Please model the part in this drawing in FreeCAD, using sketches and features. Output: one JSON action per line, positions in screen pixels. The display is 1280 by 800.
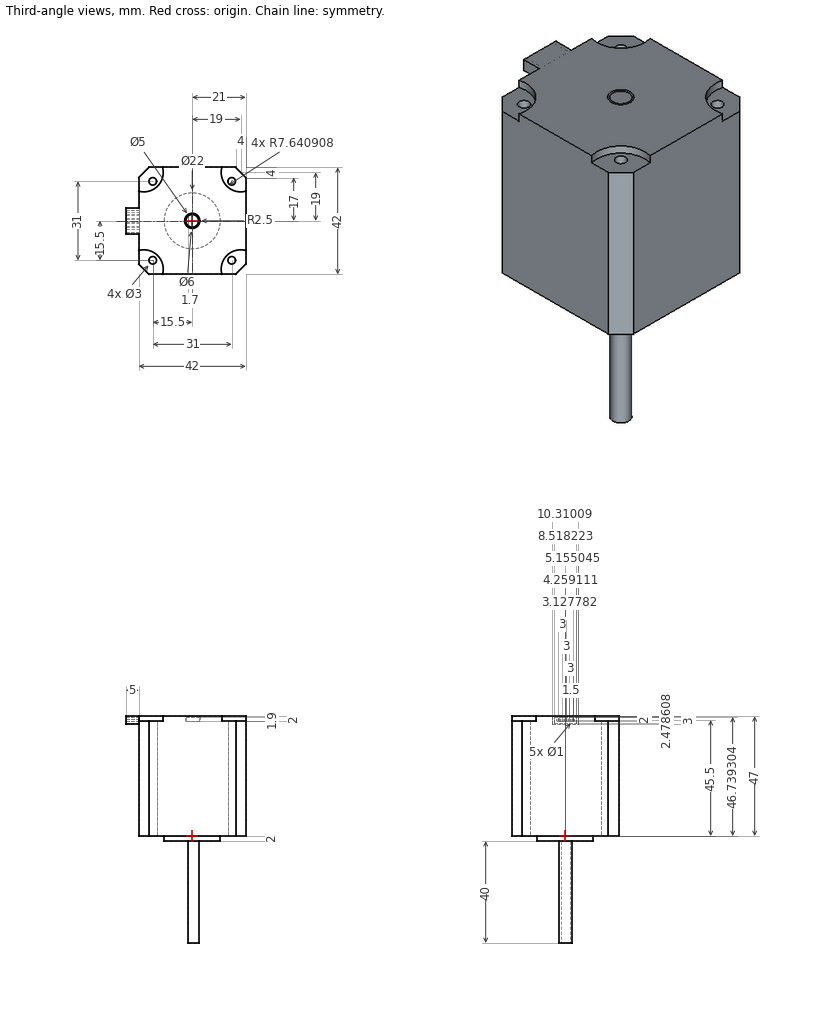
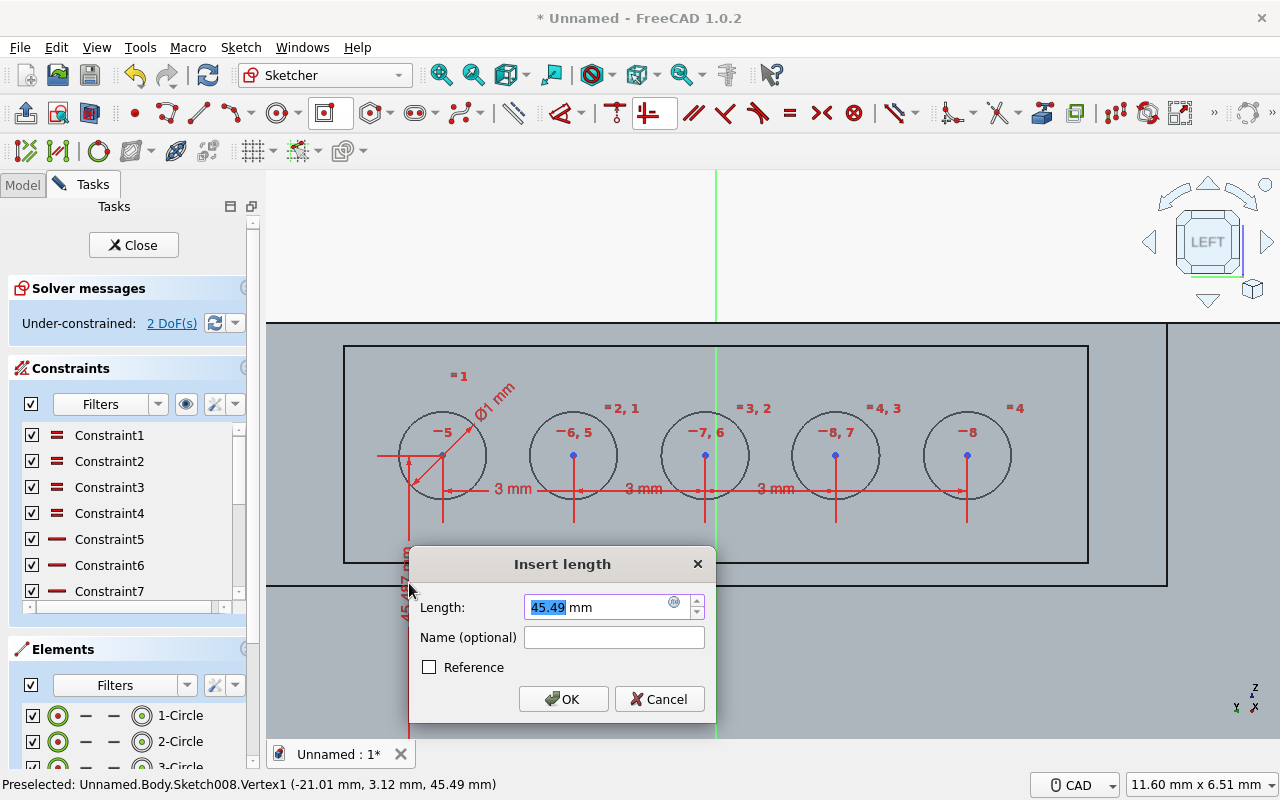
{"action": "type", "text": "45.5"}
{"action": "key", "text": "Return"}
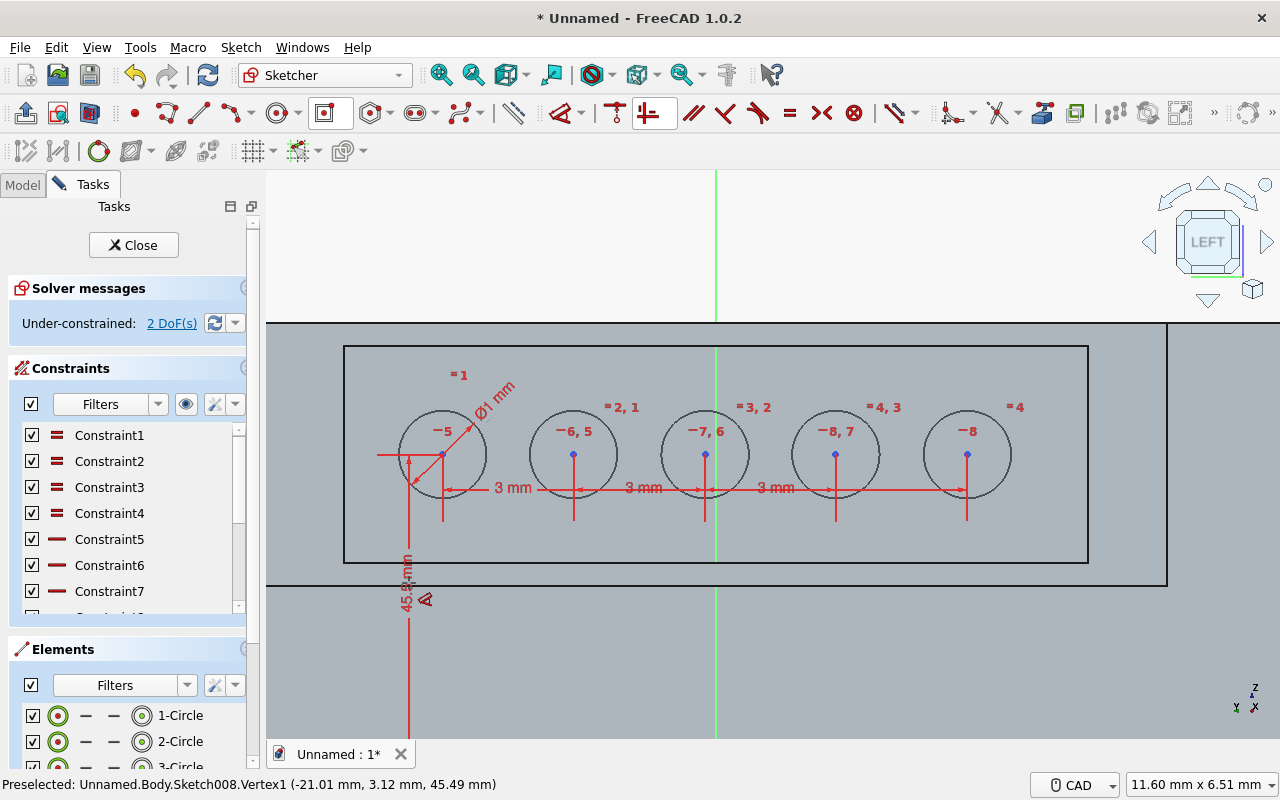
{"action": "left_click", "coordinate": [443, 455]}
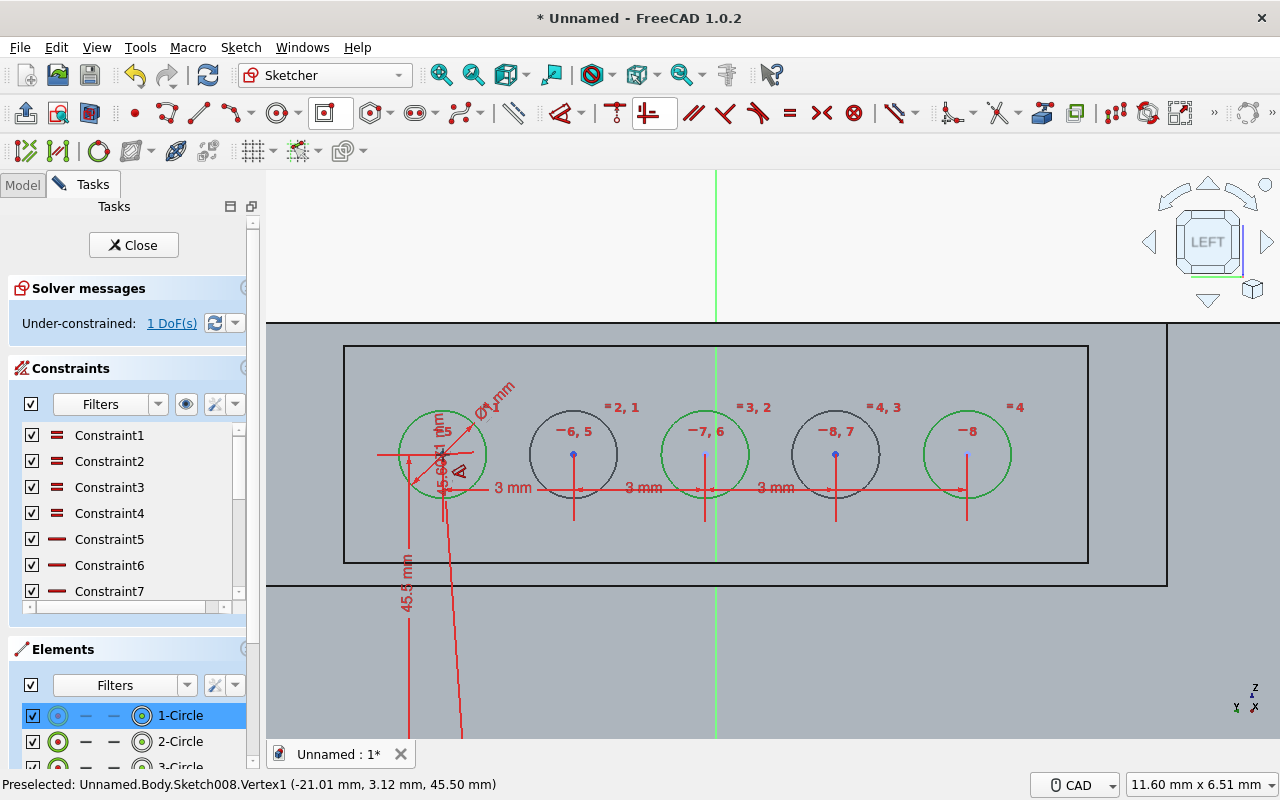
{"action": "left_click", "coordinate": [574, 455]}
{"action": "left_click", "coordinate": [508, 513]}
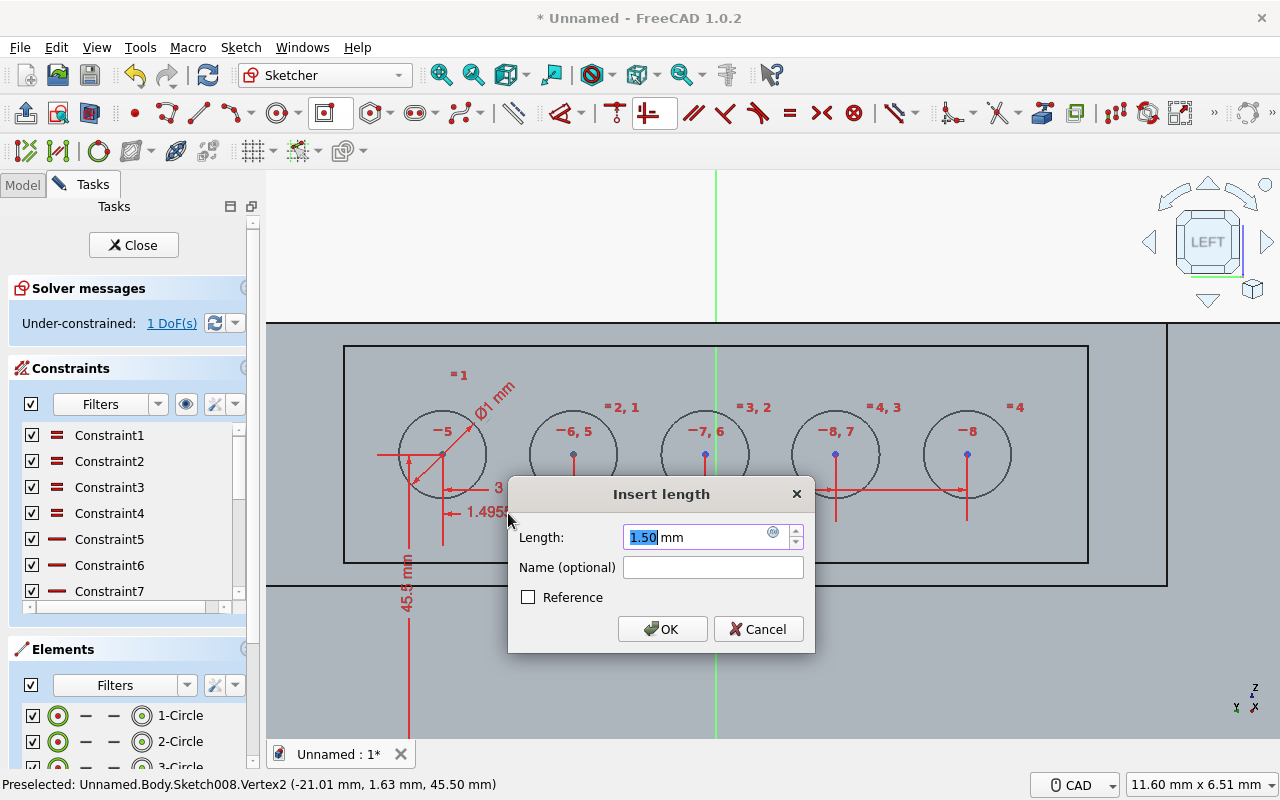
{"action": "type", "text": "1.5"}
{"action": "key", "text": "Return"}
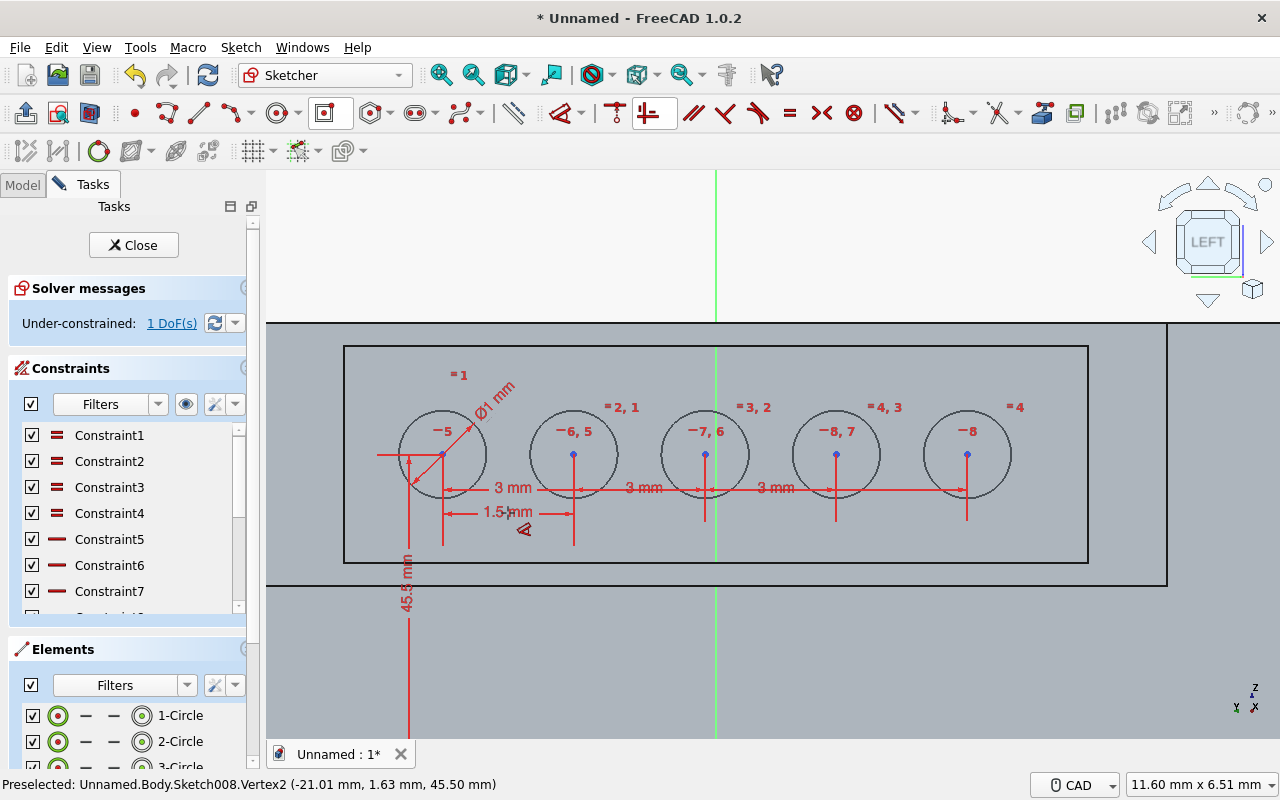
{"action": "left_click", "coordinate": [443, 455]}
{"action": "left_click", "coordinate": [642, 421]}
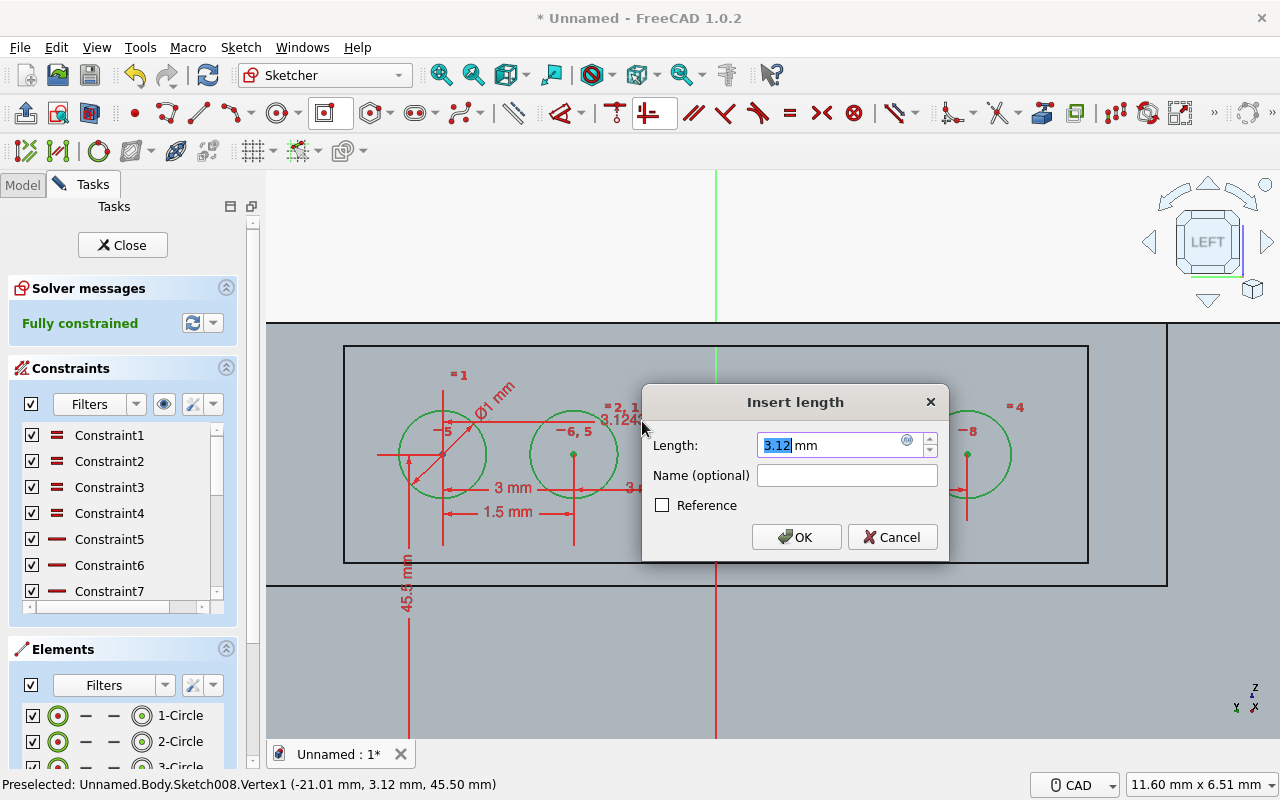
{"action": "type", "text": "3.127782"}
{"action": "key", "text": "Return"}
{"action": "key", "text": "Escape"}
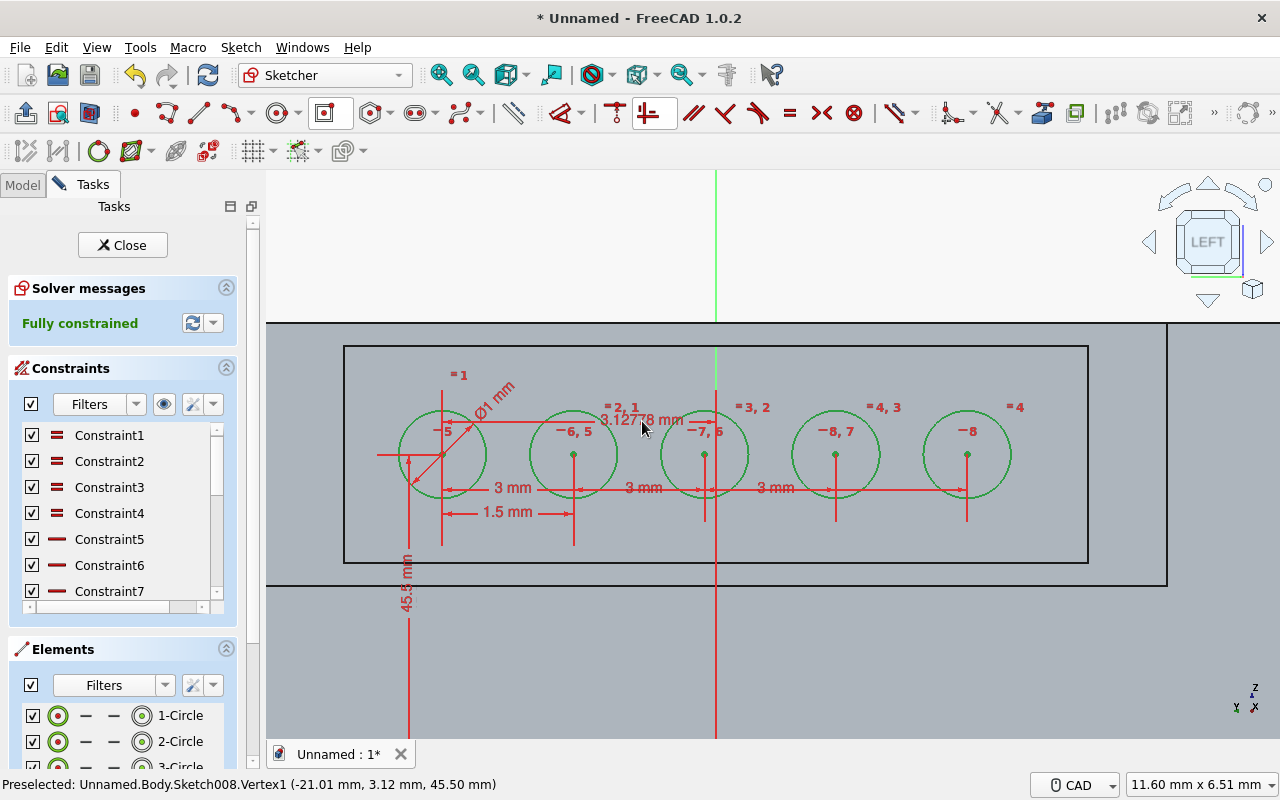
{"action": "left_click", "coordinate": [123, 245]}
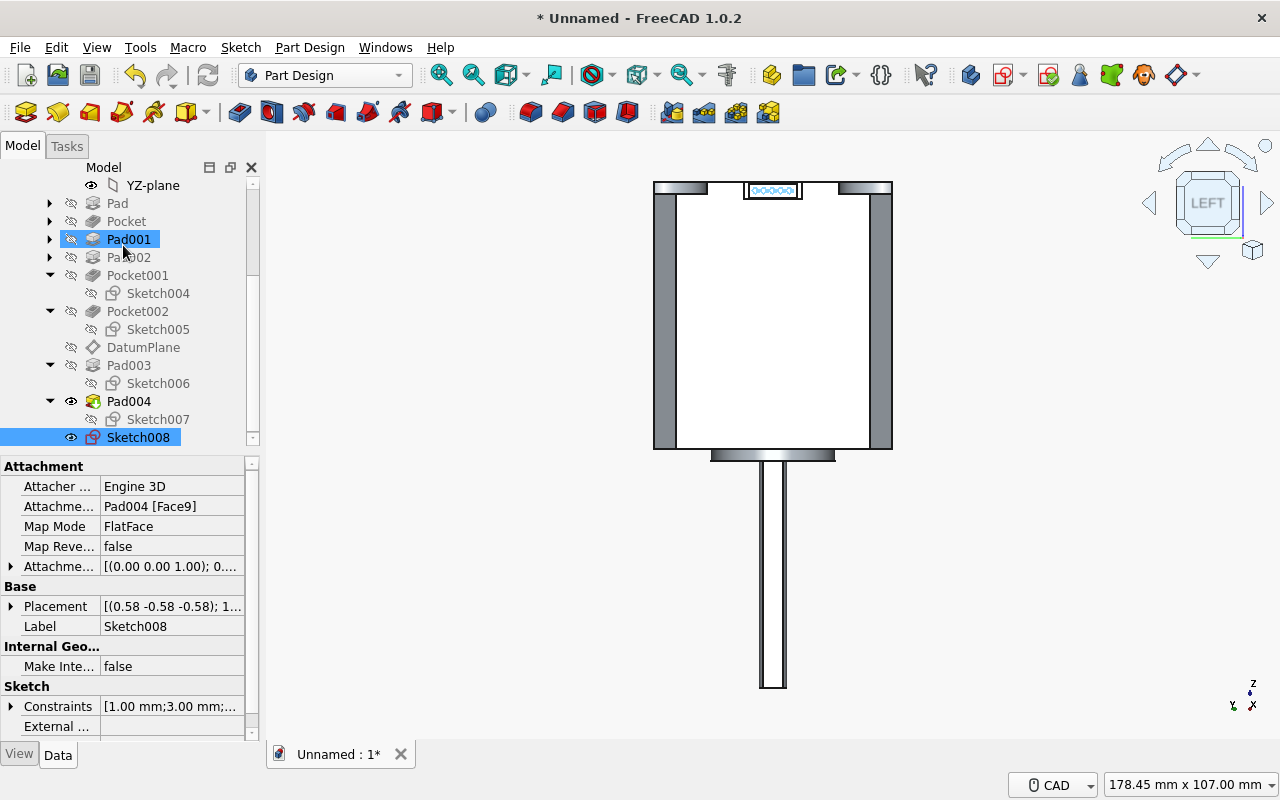
{"action": "left_click", "coordinate": [26, 112]}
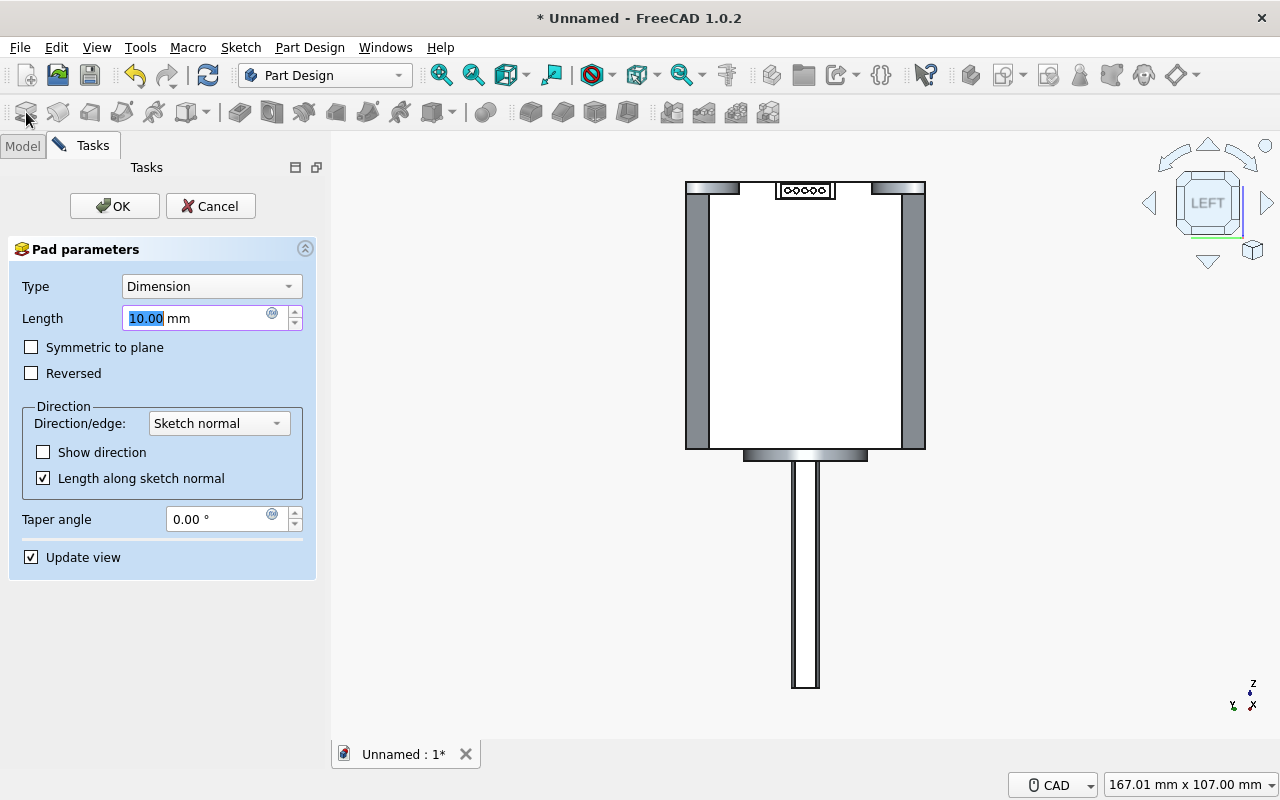
{"action": "type", "text": "5"}
{"action": "key", "text": "Tab"}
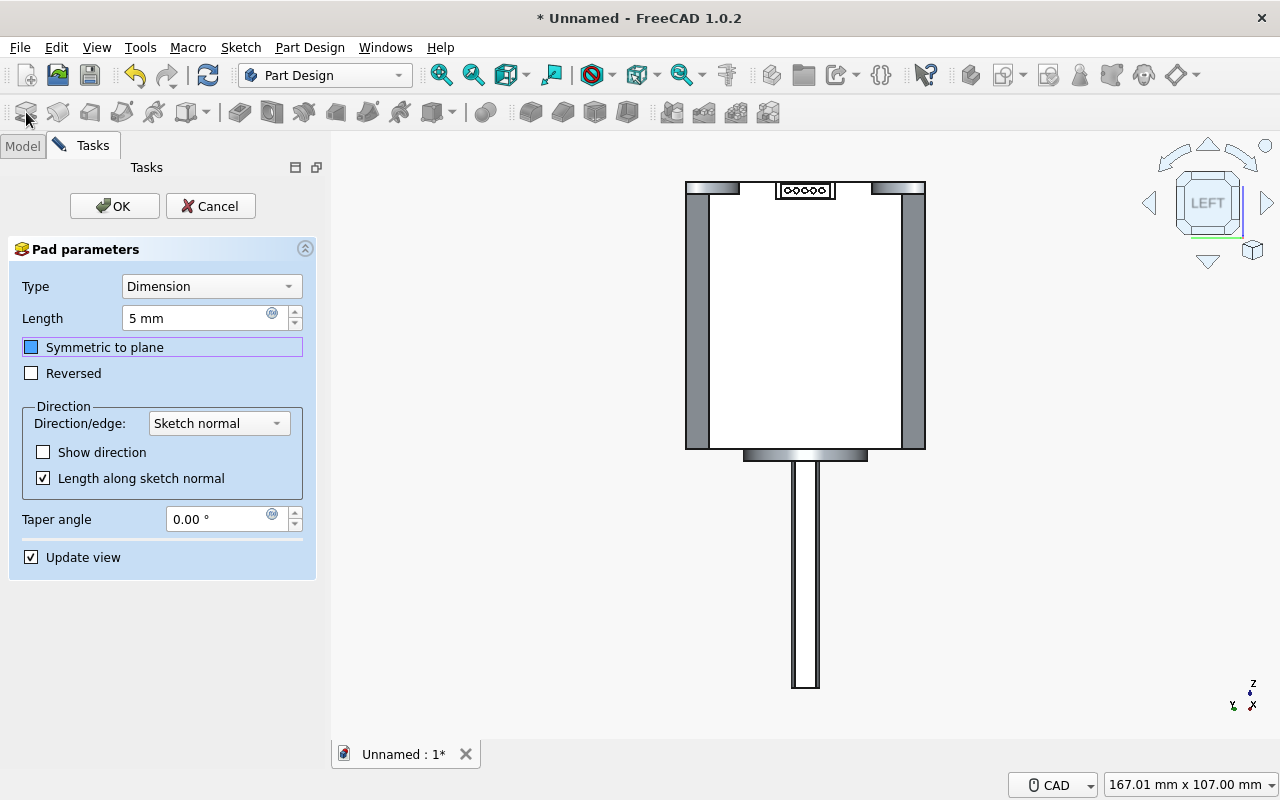
{"action": "left_click", "coordinate": [115, 206]}